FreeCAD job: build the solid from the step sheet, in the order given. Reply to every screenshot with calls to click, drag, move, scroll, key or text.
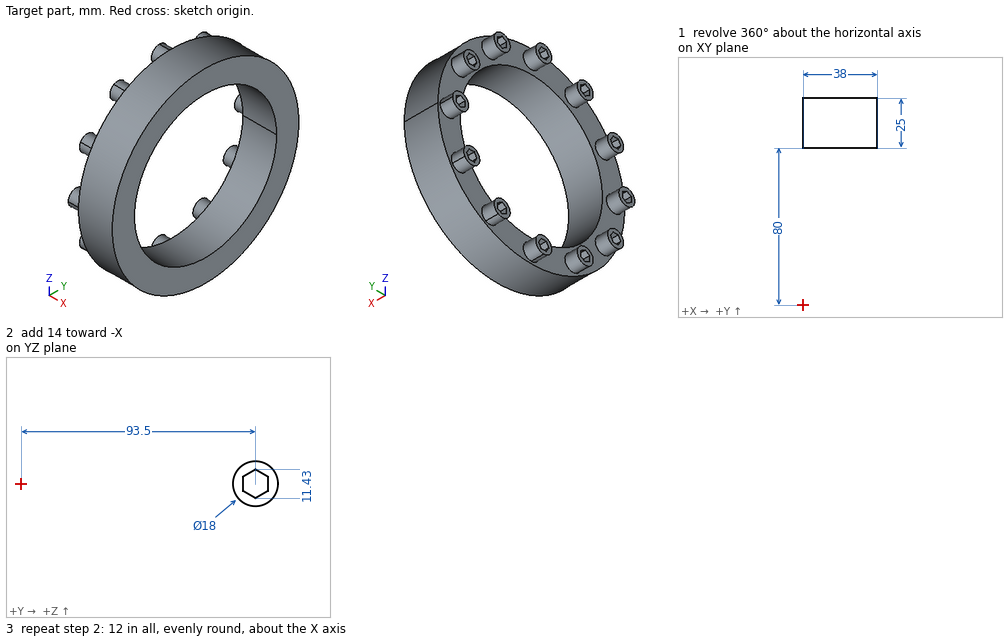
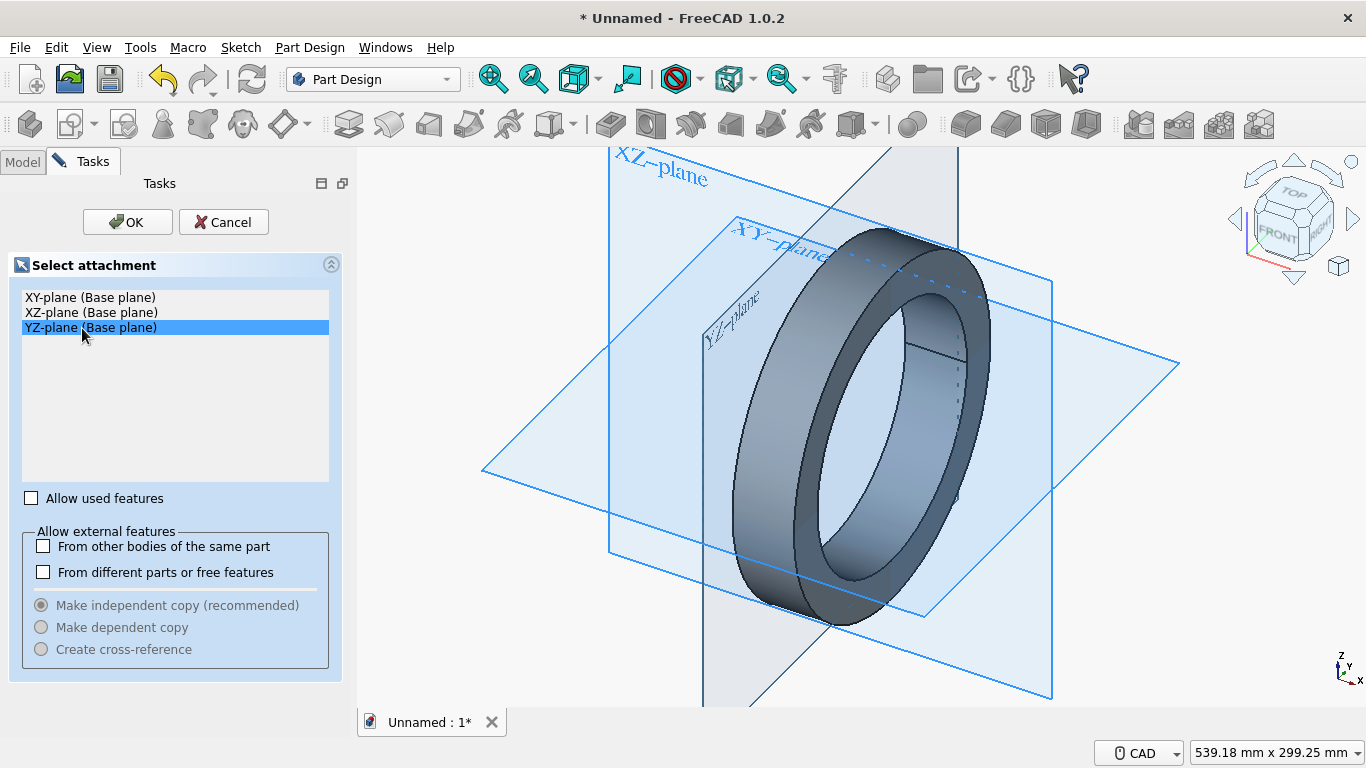
click(128, 222)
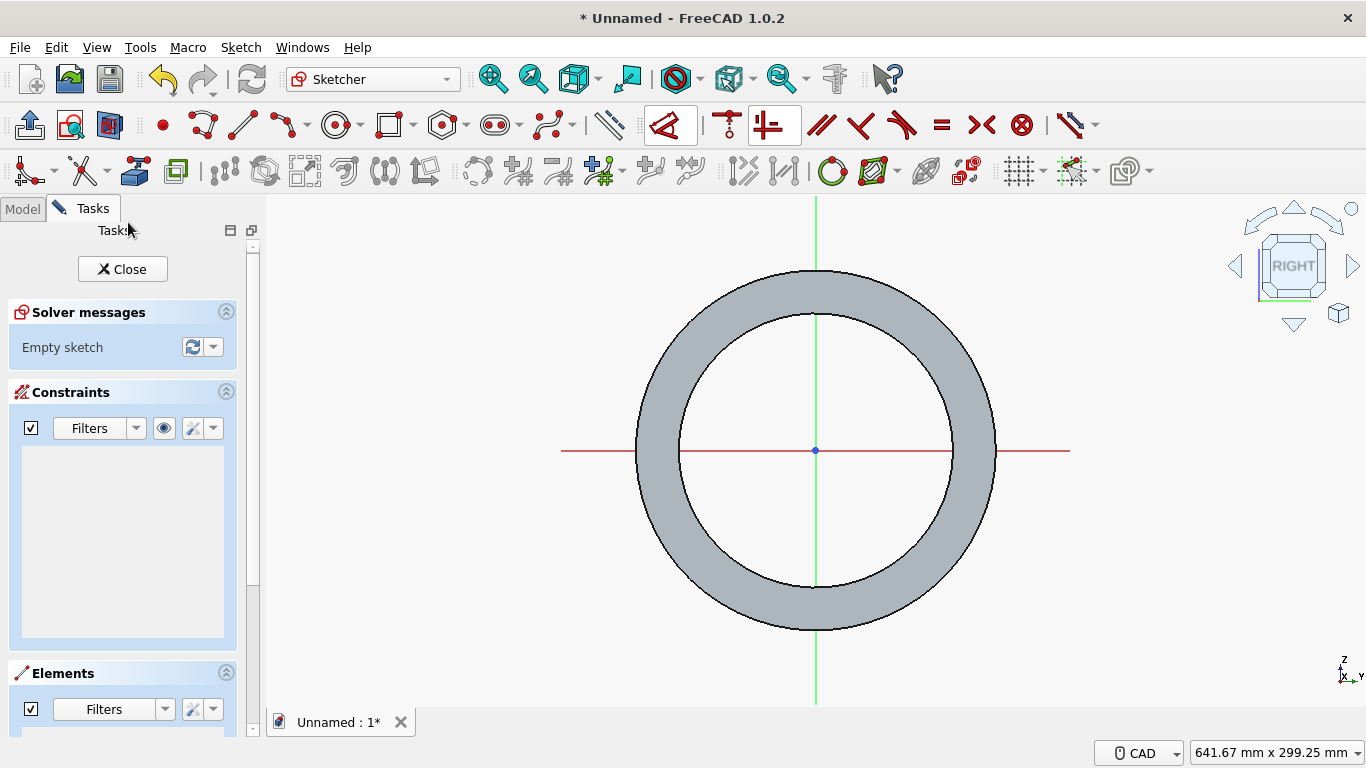
click(110, 126)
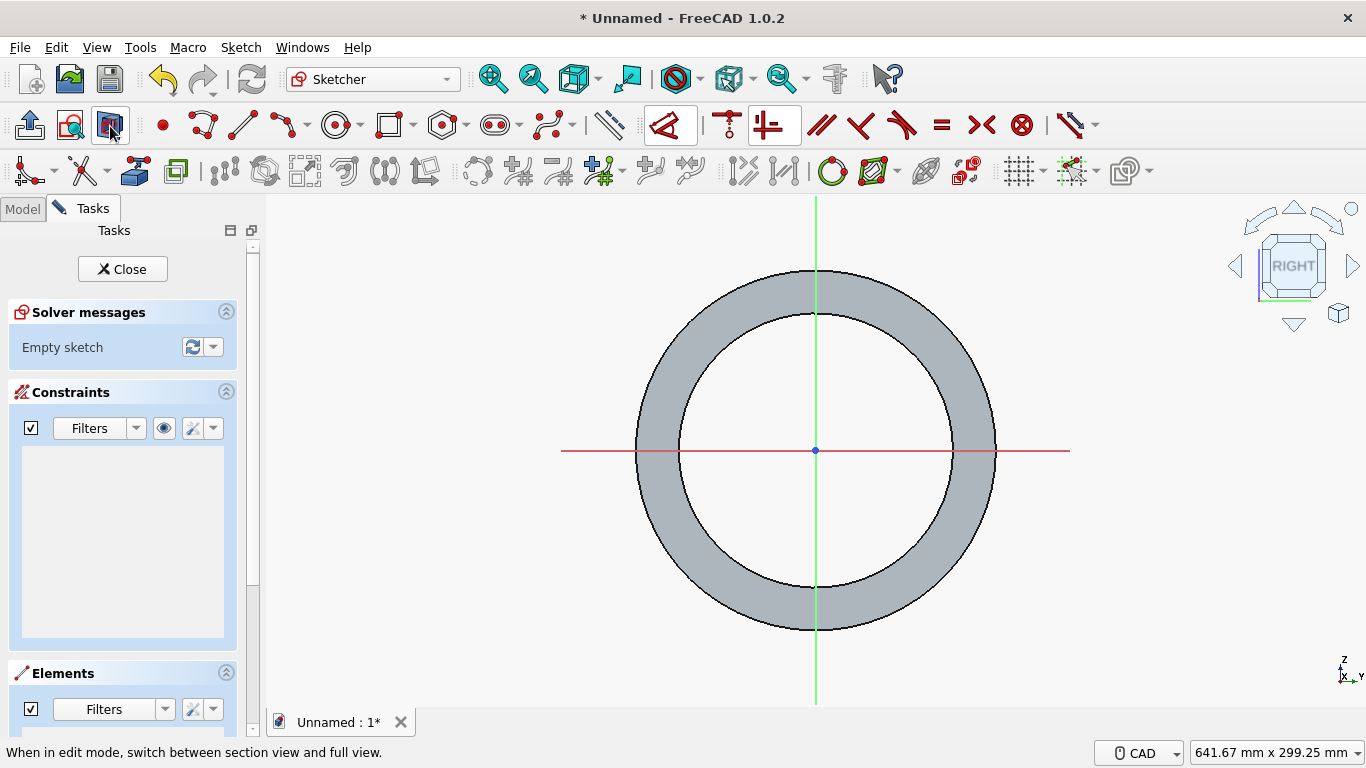
scroll(999, 450, up, 12)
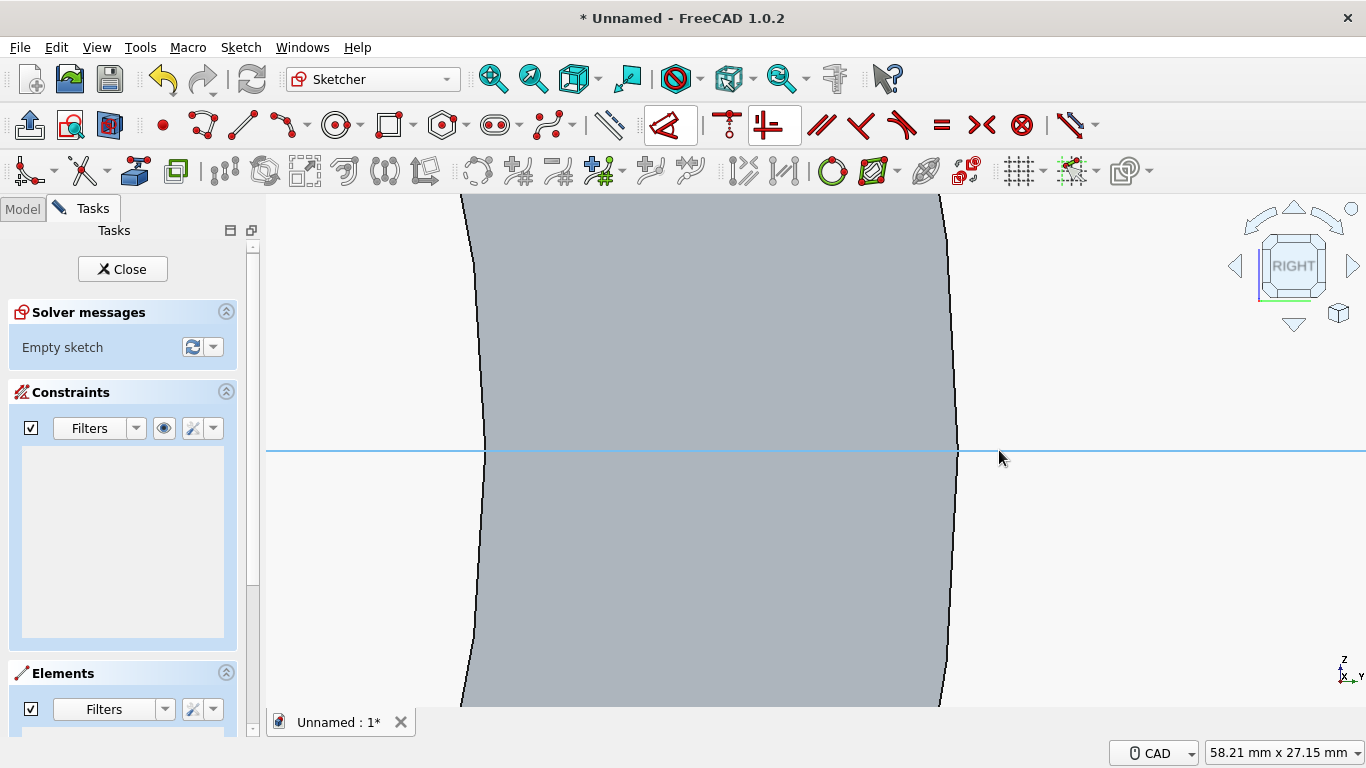
click(442, 126)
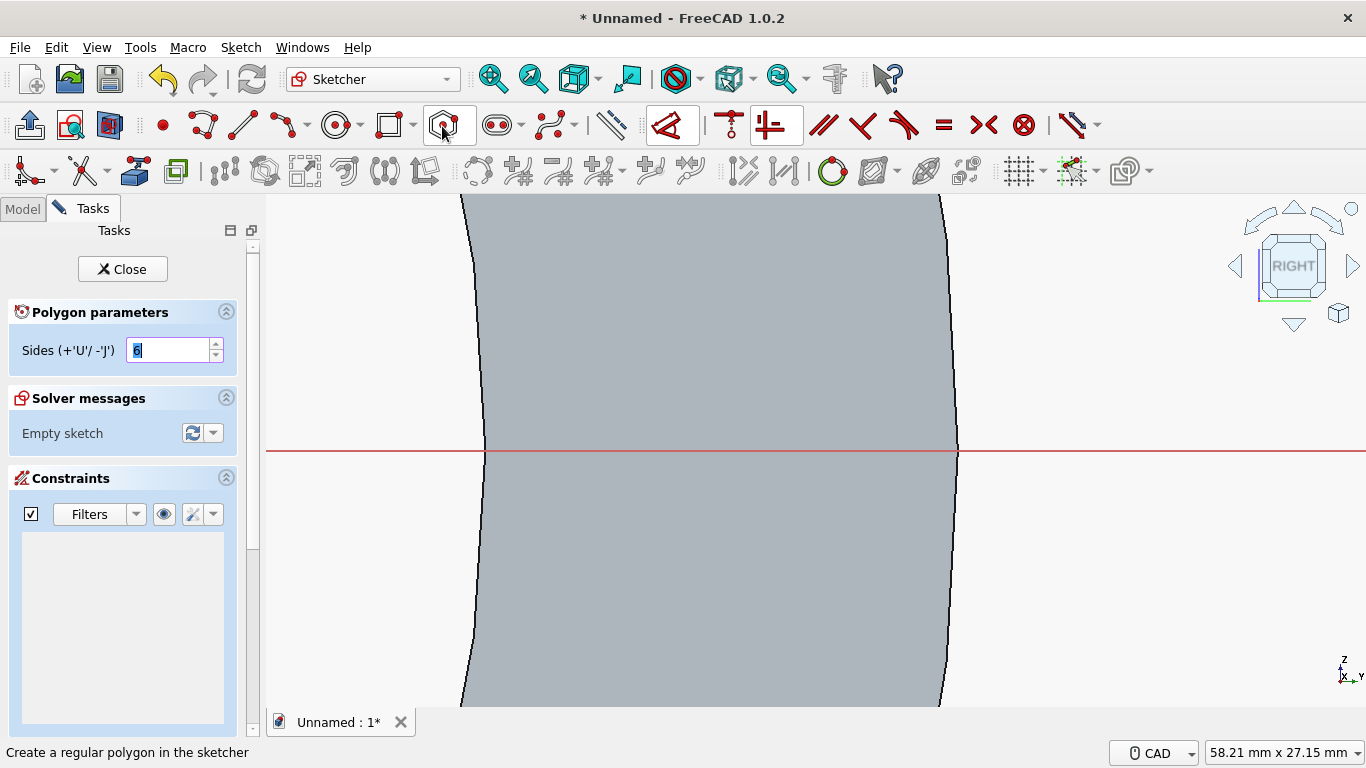
click(741, 450)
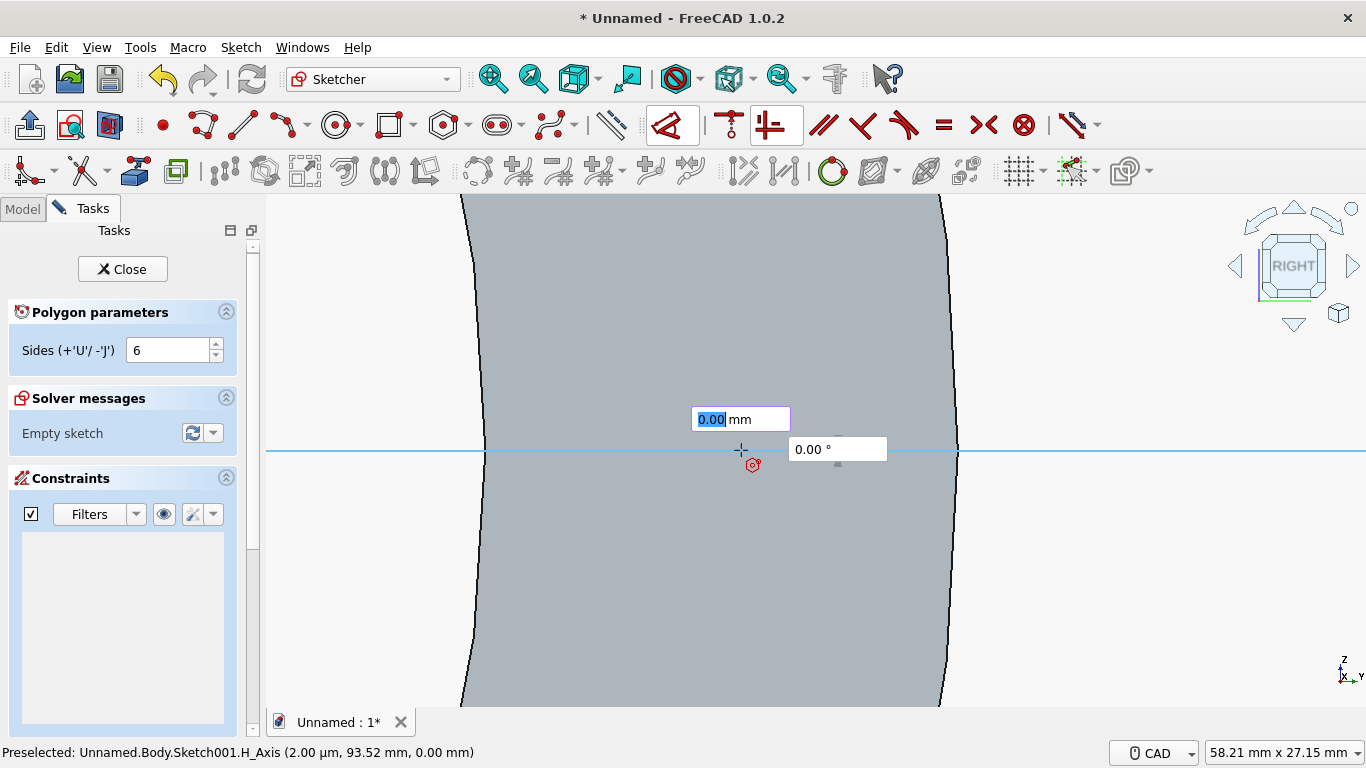
click(741, 343)
key(Escape)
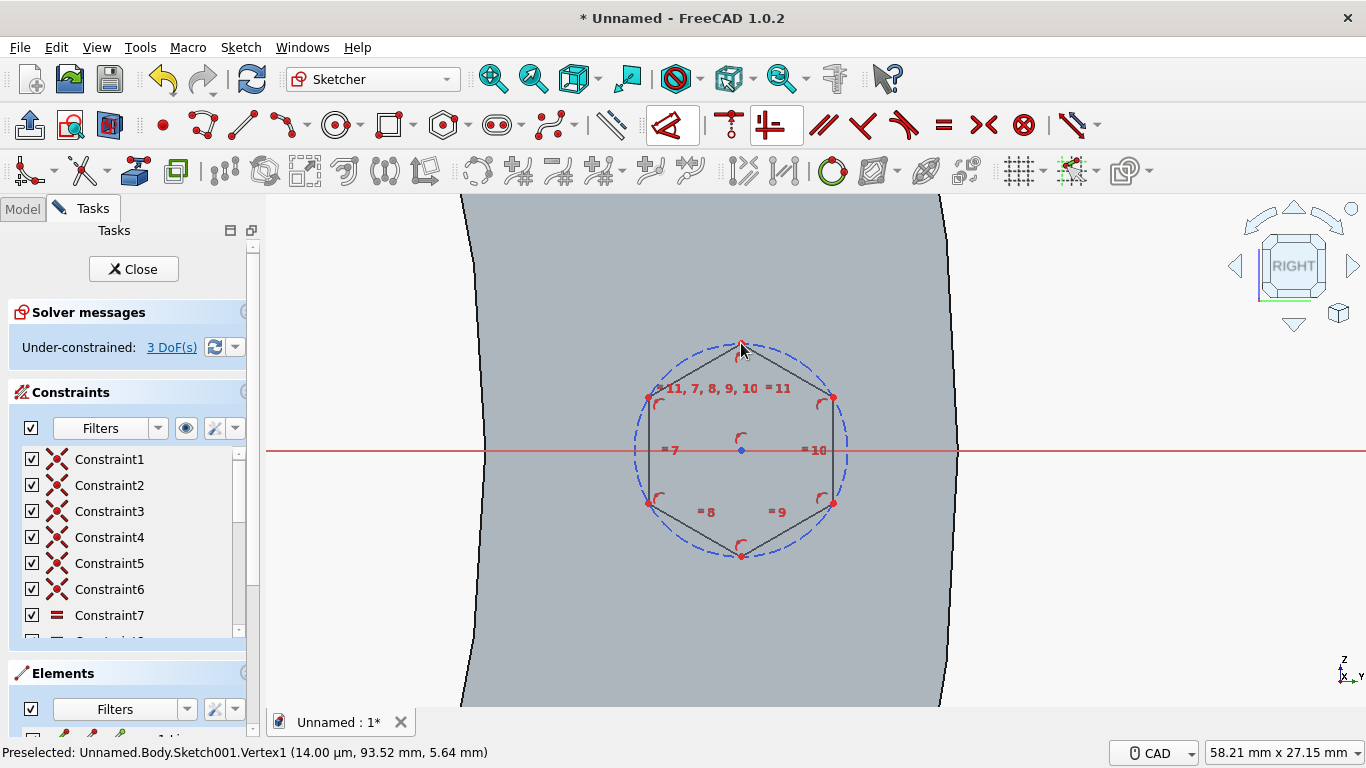
key(g)
key(c)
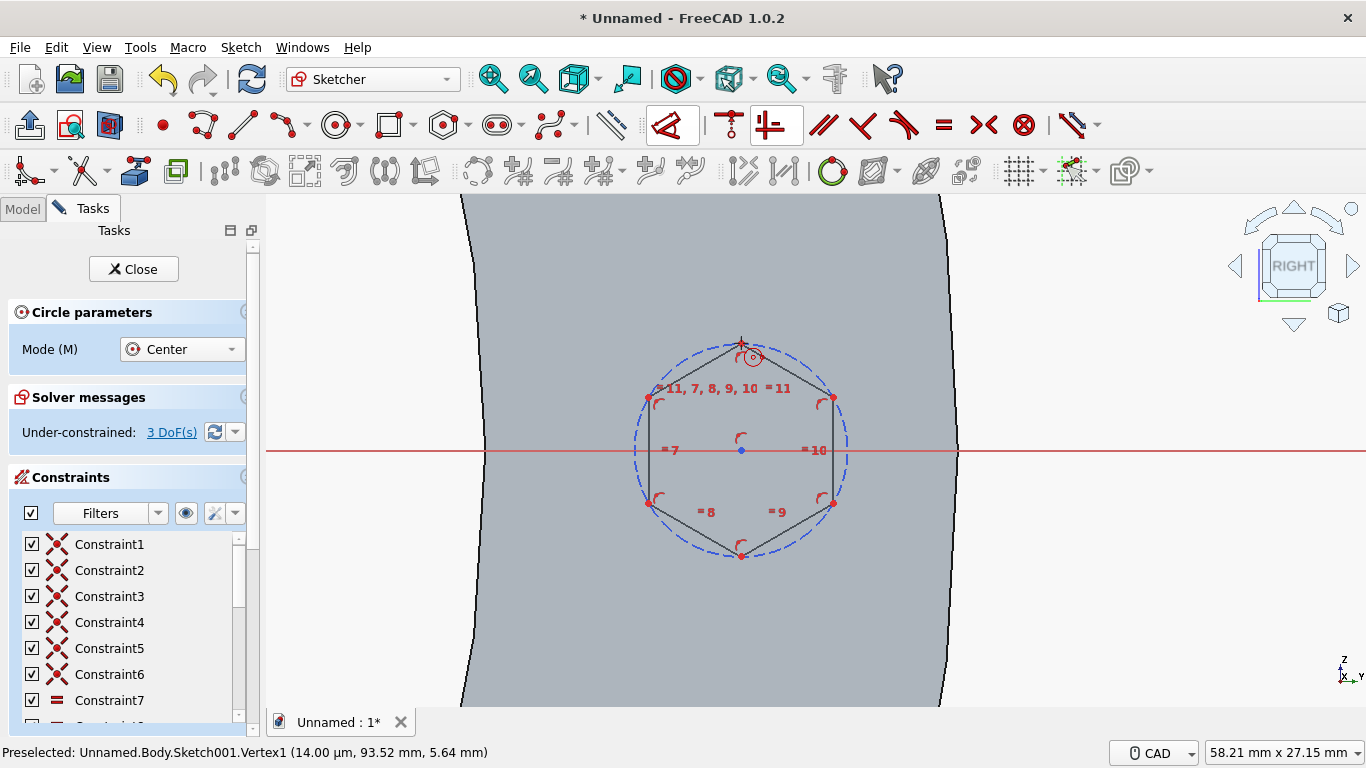
click(741, 450)
move(861, 330)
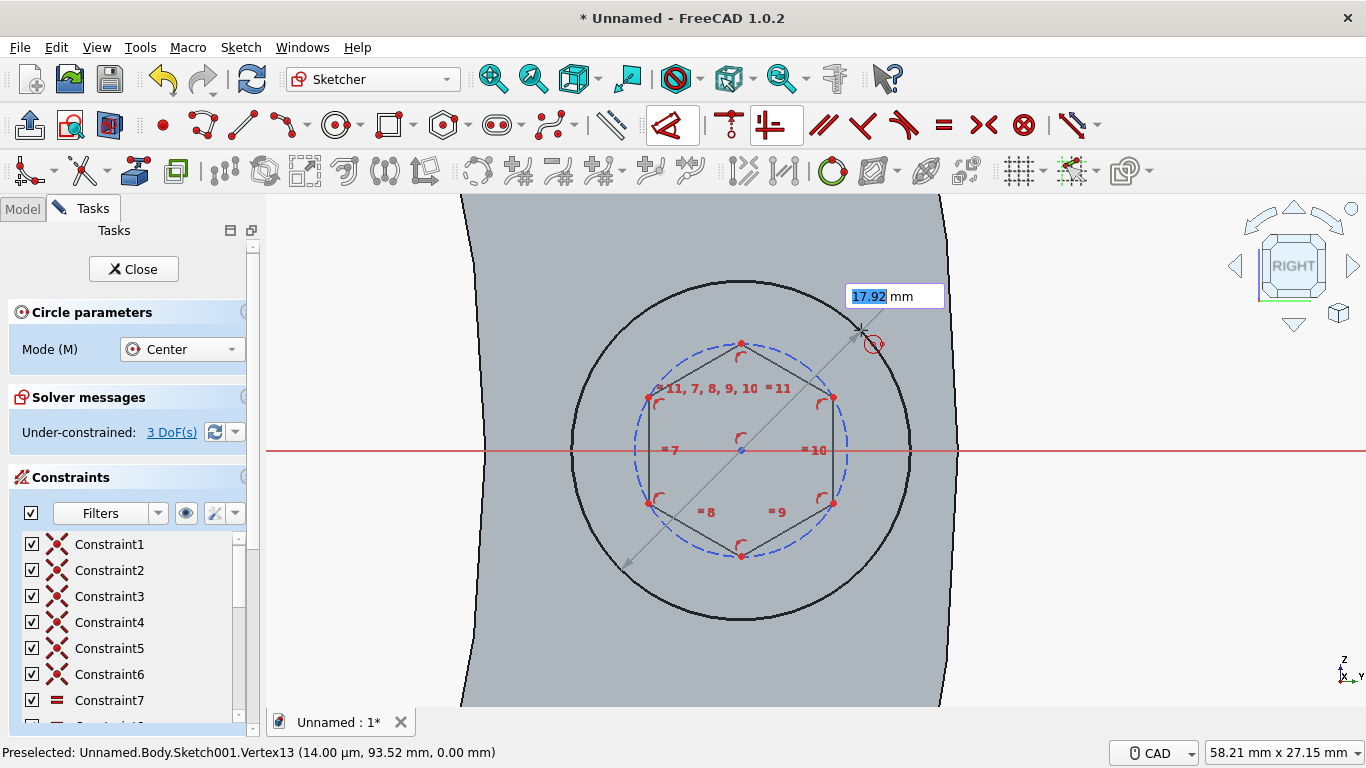
text(18)
key(Return)
key(Escape)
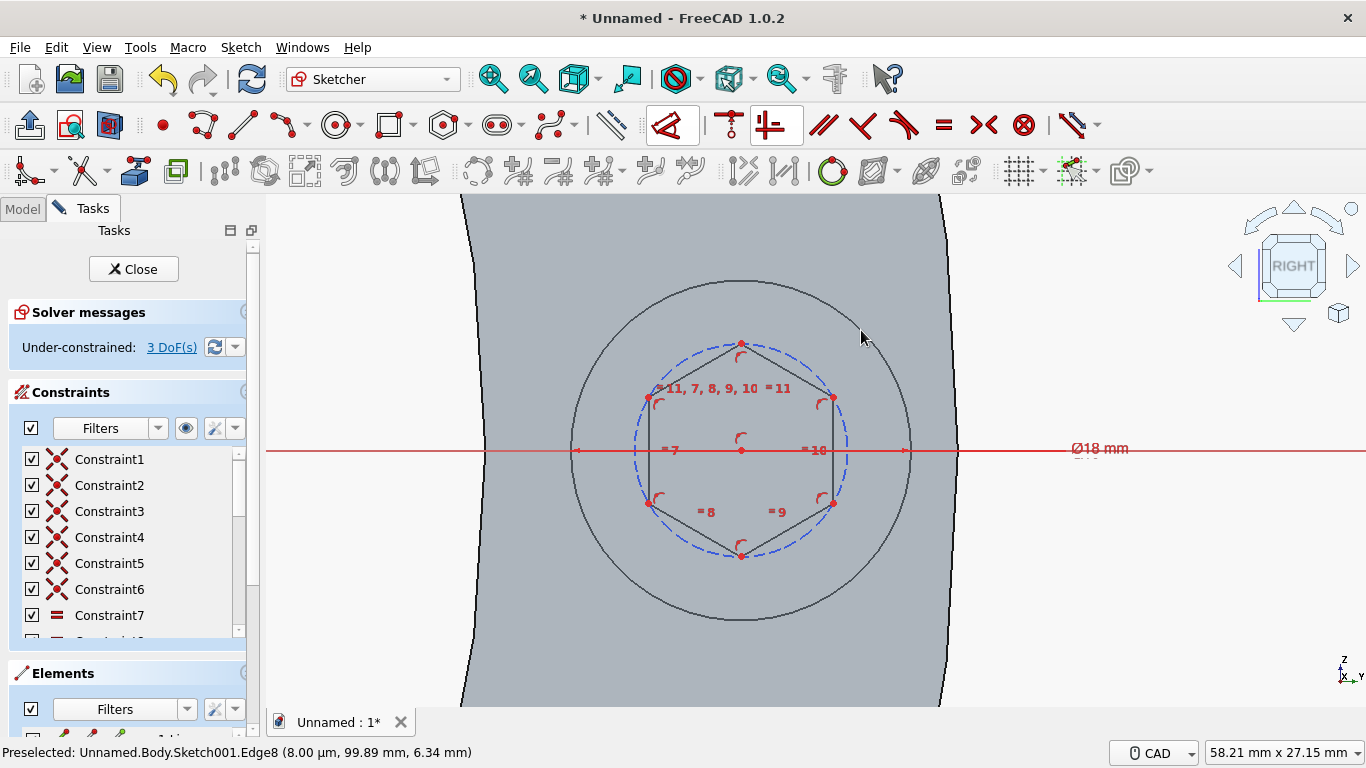
click(649, 429)